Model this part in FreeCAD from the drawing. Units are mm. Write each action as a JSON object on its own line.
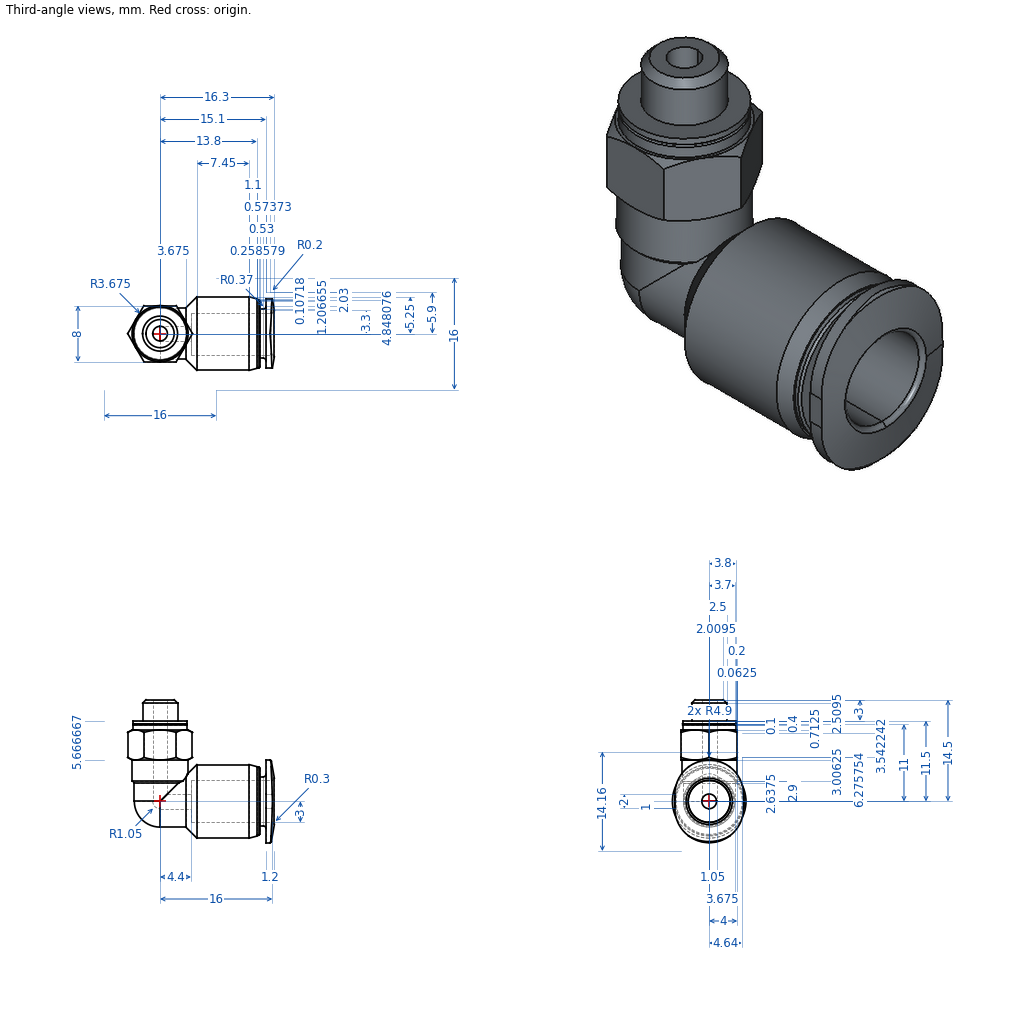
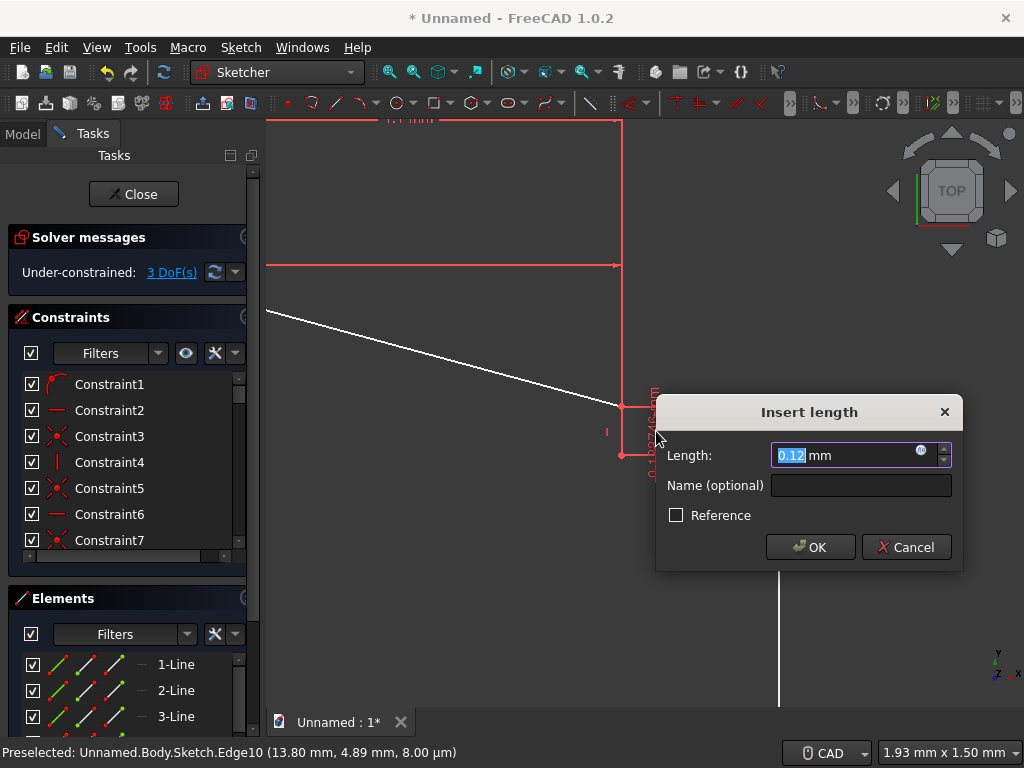
{"action": "type", "text": "0.10718"}
{"action": "key", "text": "Return"}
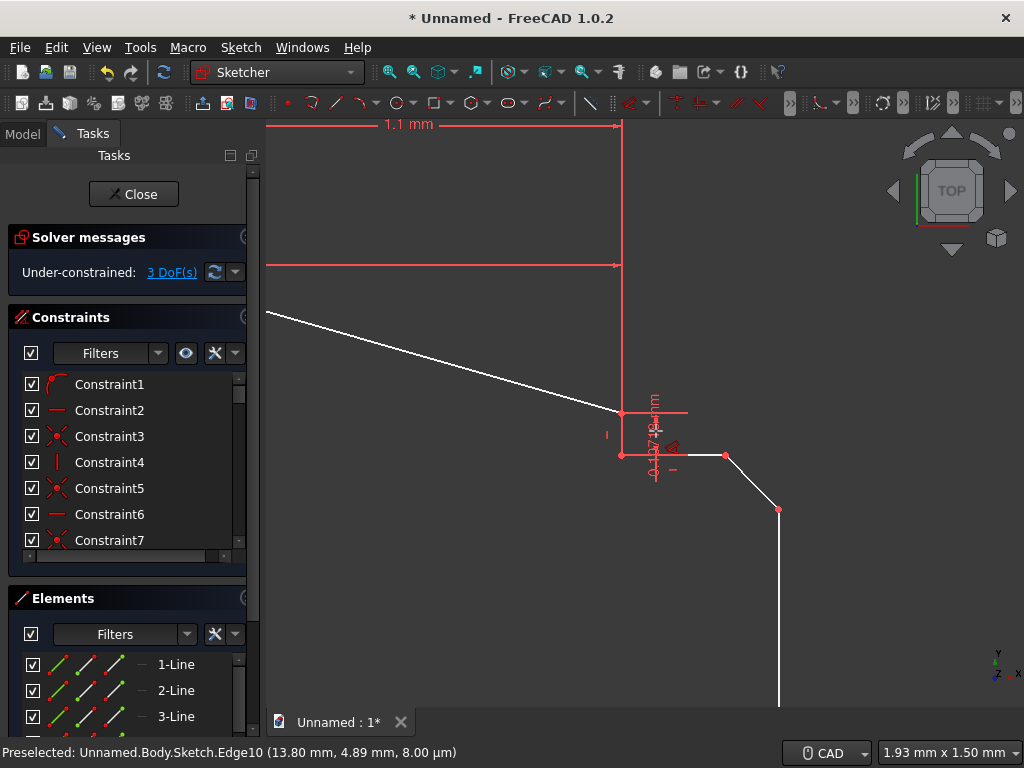
{"action": "scroll", "coordinate": [728, 372], "scroll_direction": "down", "scroll_amount": 15}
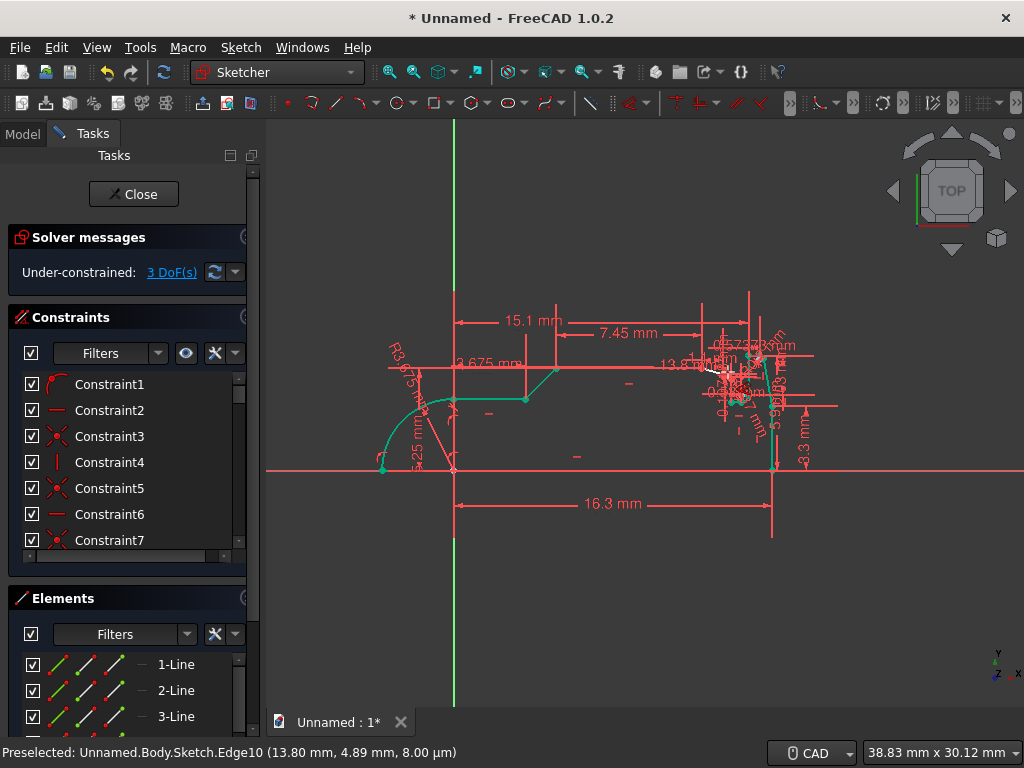
{"action": "scroll", "coordinate": [731, 386], "scroll_direction": "up", "scroll_amount": 4}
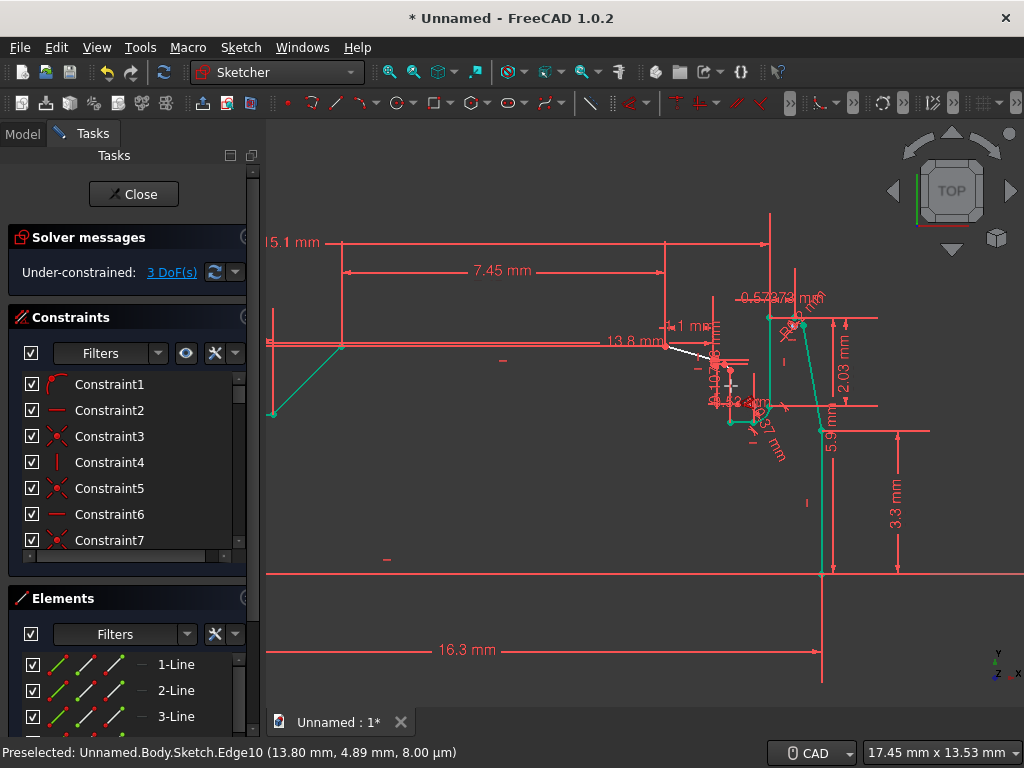
{"action": "left_click", "coordinate": [730, 386]}
{"action": "left_click", "coordinate": [696, 384]}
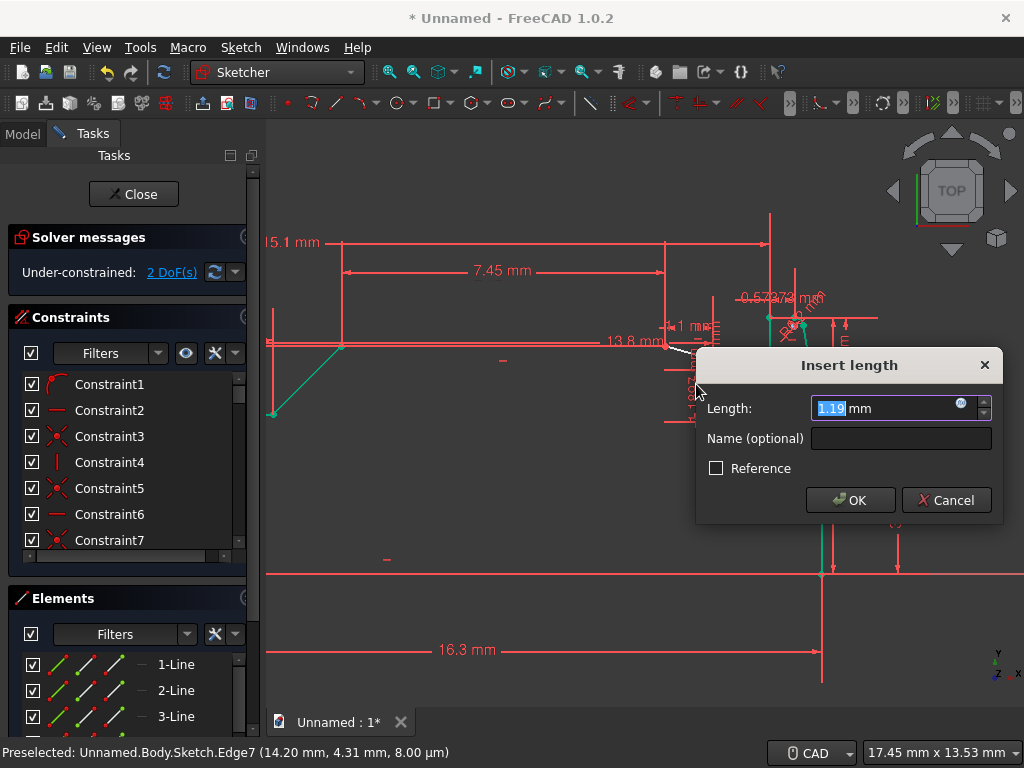
{"action": "type", "text": "1.206655"}
{"action": "key", "text": "Return"}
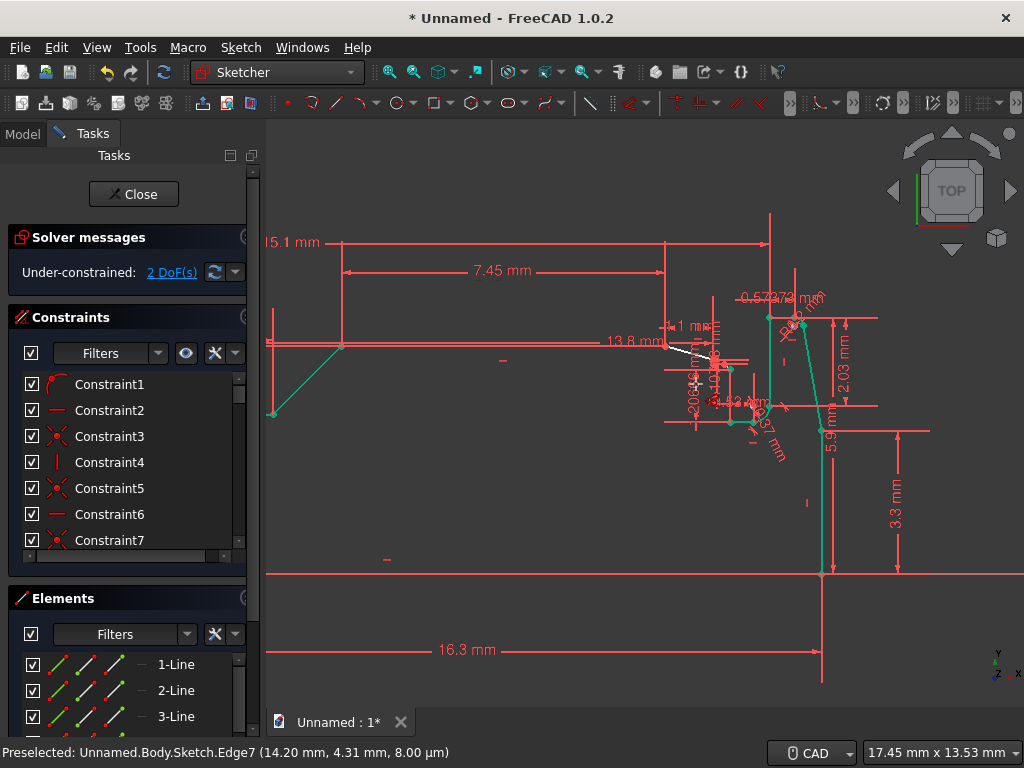
{"action": "scroll", "coordinate": [719, 364], "scroll_direction": "up", "scroll_amount": 7}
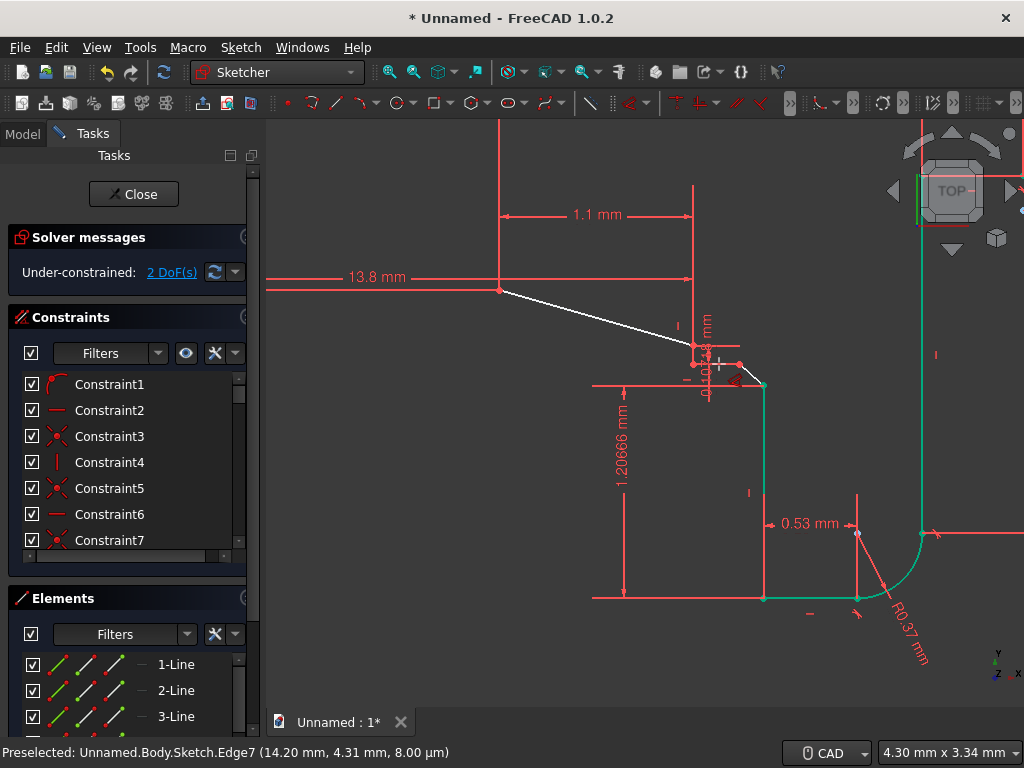
{"action": "left_click", "coordinate": [717, 364]}
{"action": "left_click", "coordinate": [717, 330]}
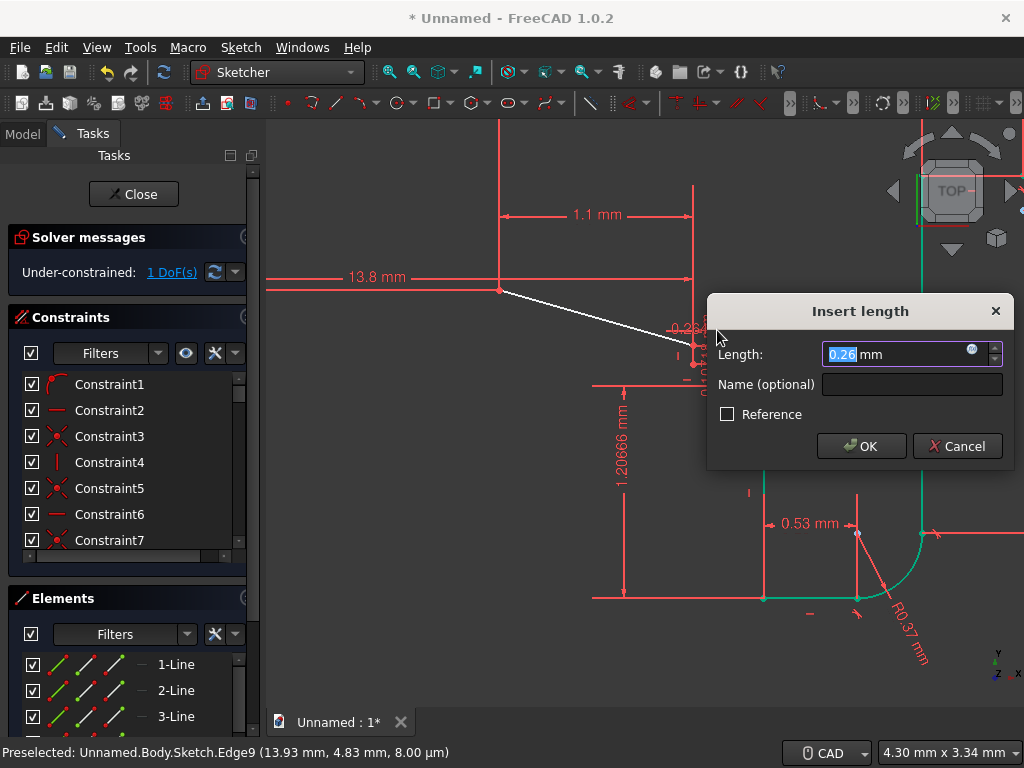
{"action": "type", "text": "0.258579"}
{"action": "key", "text": "Return"}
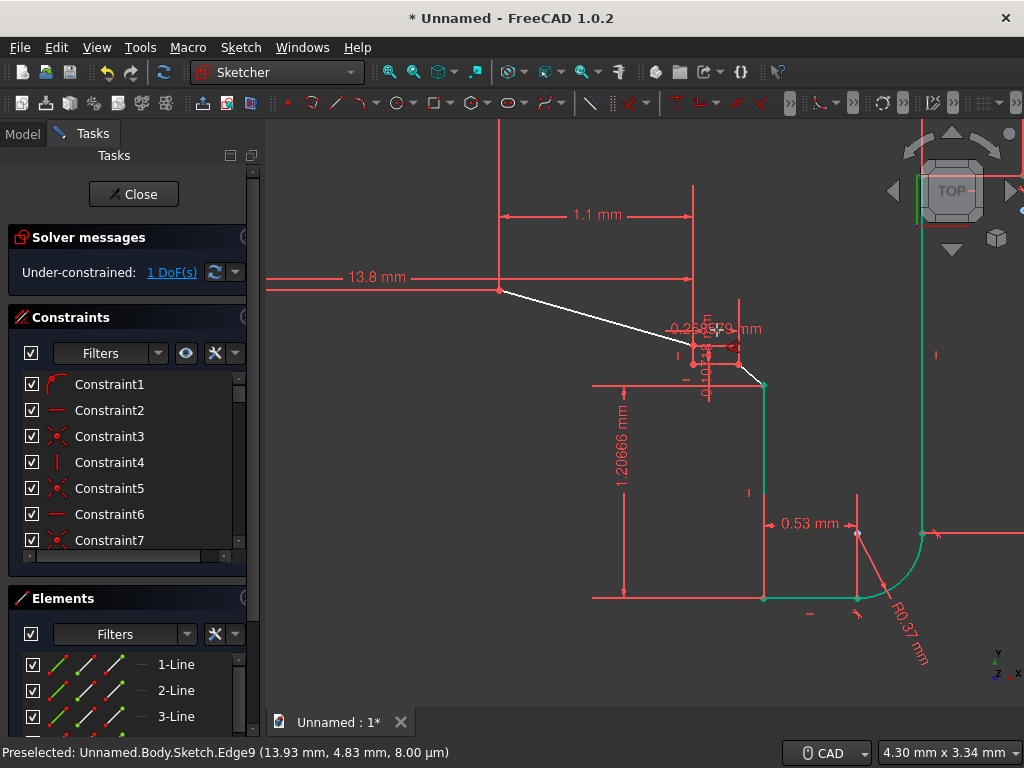
{"action": "left_click", "coordinate": [739, 364]}
{"action": "left_click", "coordinate": [773, 632]}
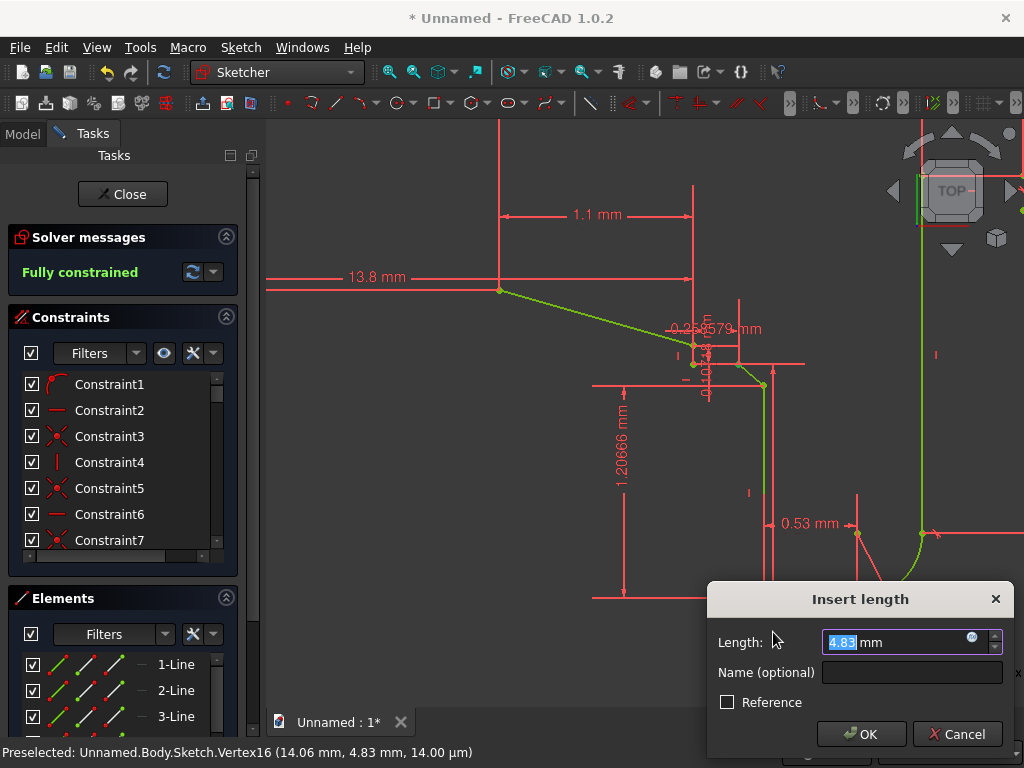
{"action": "type", "text": "4.848076"}
{"action": "key", "text": "Return"}
{"action": "key", "text": "Escape"}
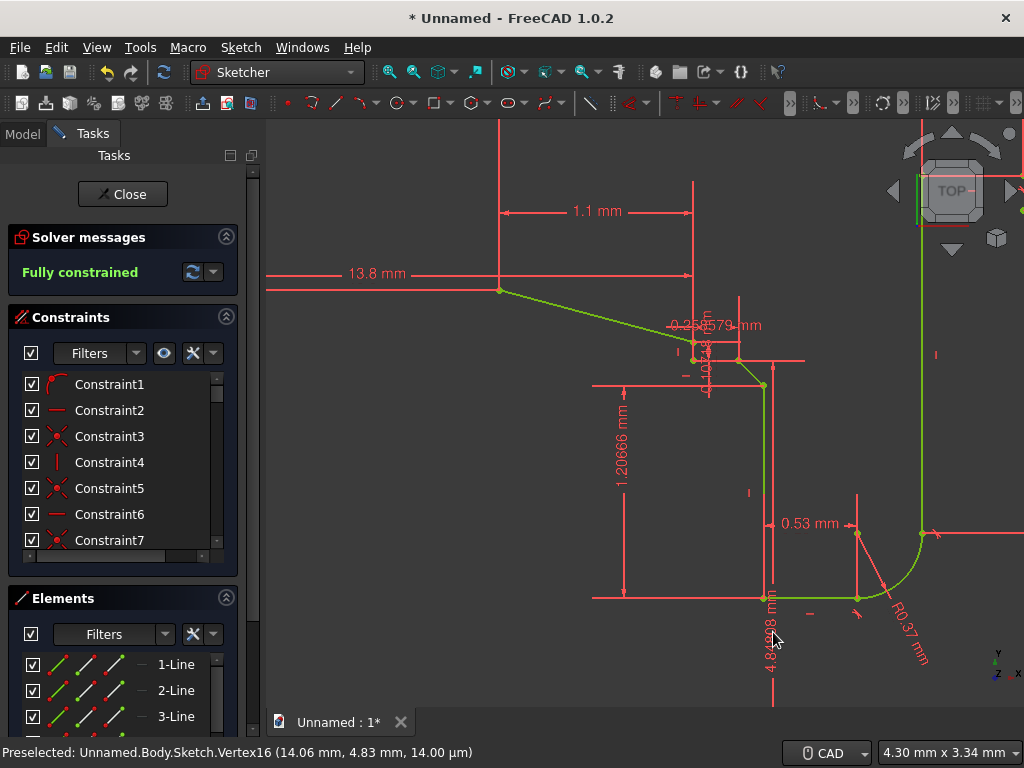
{"action": "left_click", "coordinate": [123, 194]}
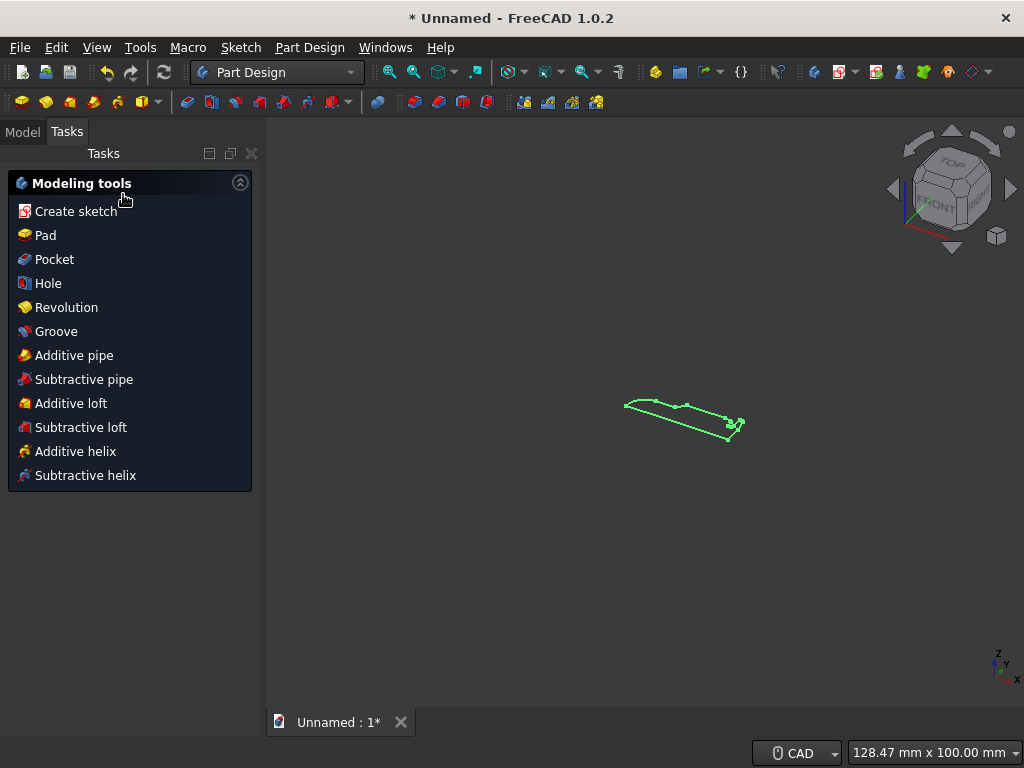
{"action": "left_click", "coordinate": [46, 102]}